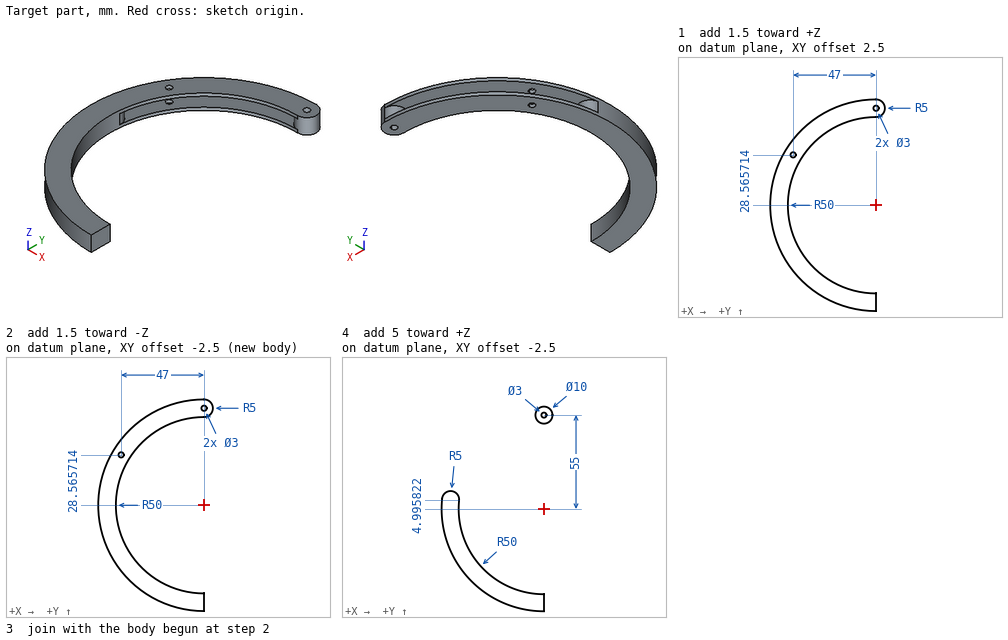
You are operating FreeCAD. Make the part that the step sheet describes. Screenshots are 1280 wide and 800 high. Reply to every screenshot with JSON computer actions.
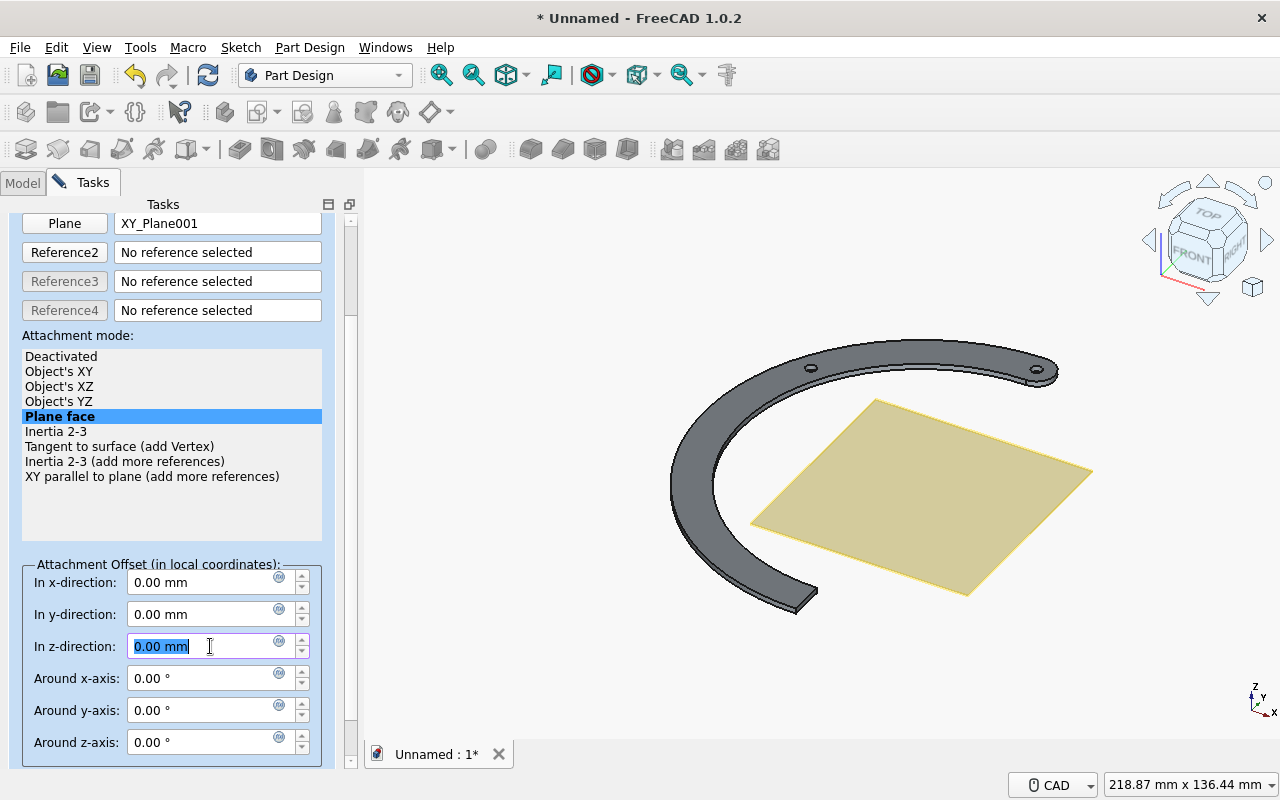
{"action": "type", "text": "-2.5"}
{"action": "key", "text": "Tab"}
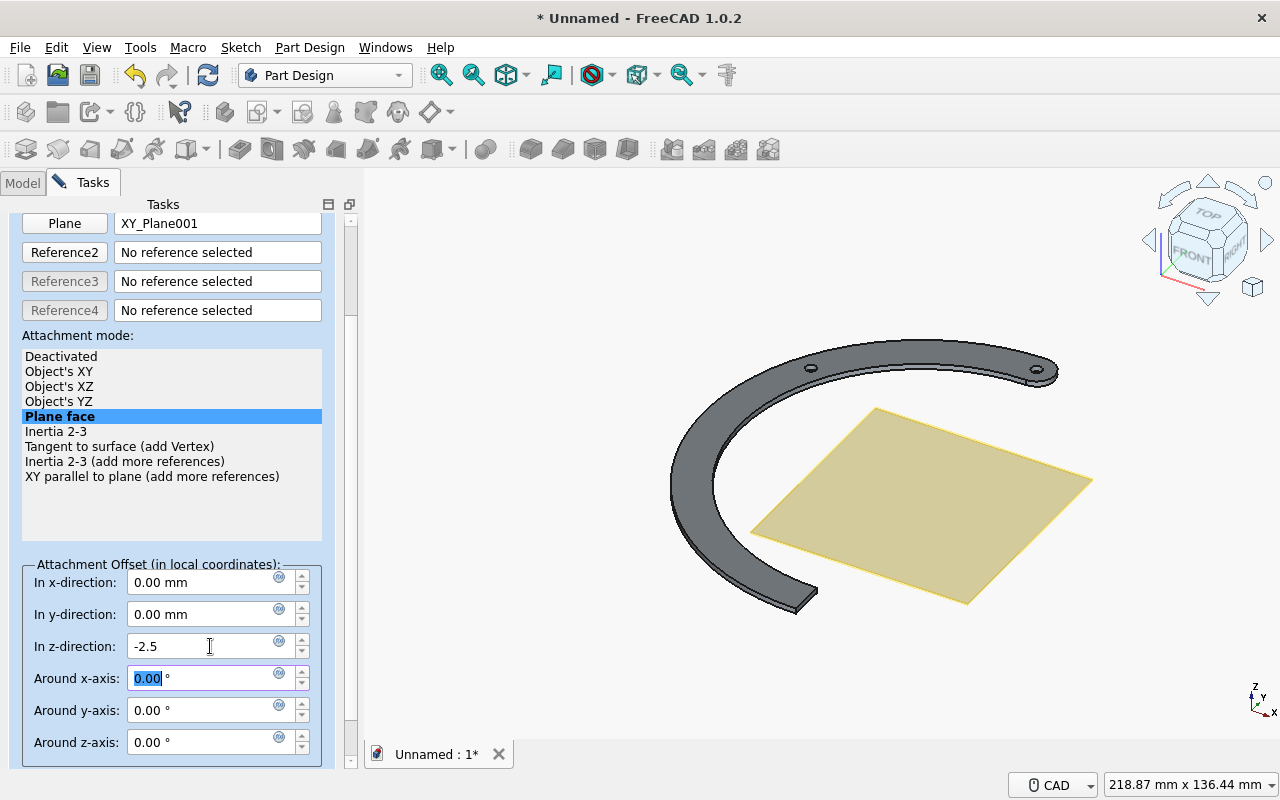
{"action": "scroll", "coordinate": [351, 491], "scroll_direction": "up", "scroll_amount": 3}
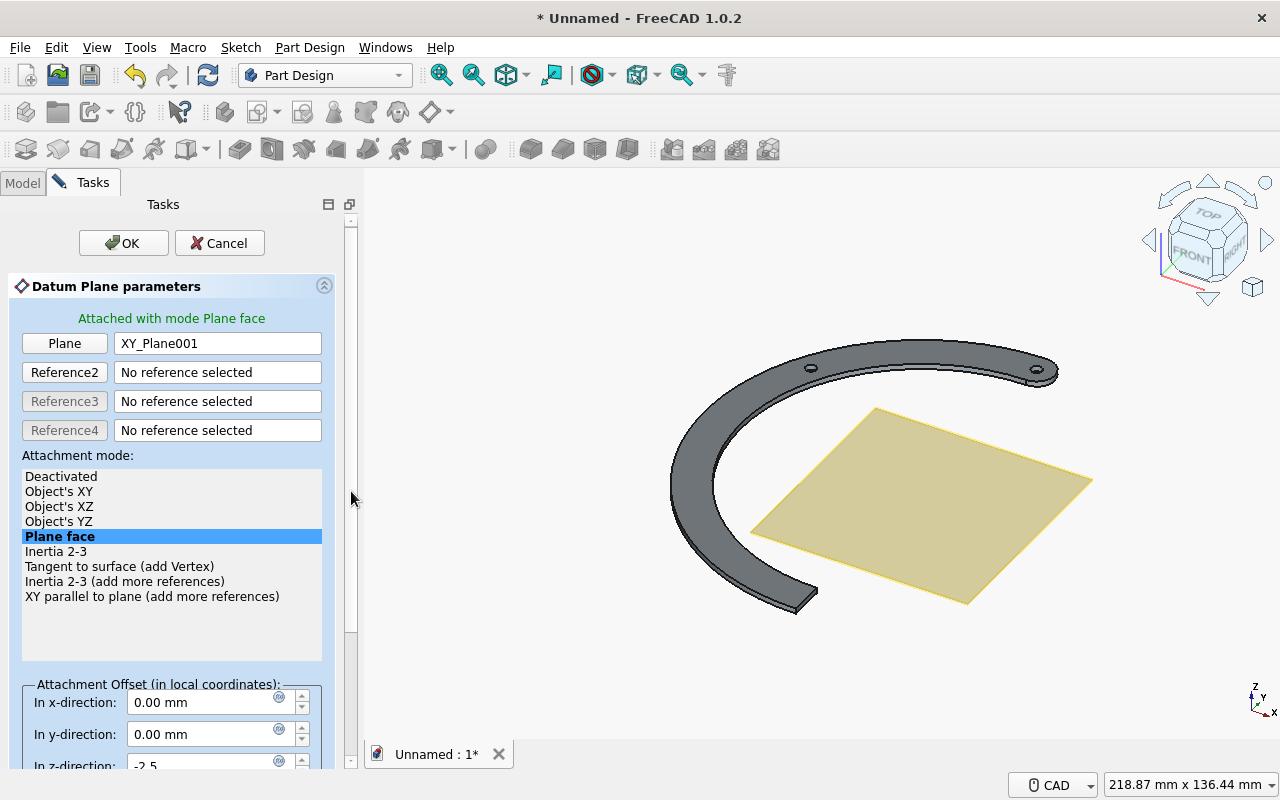
{"action": "left_click", "coordinate": [124, 243]}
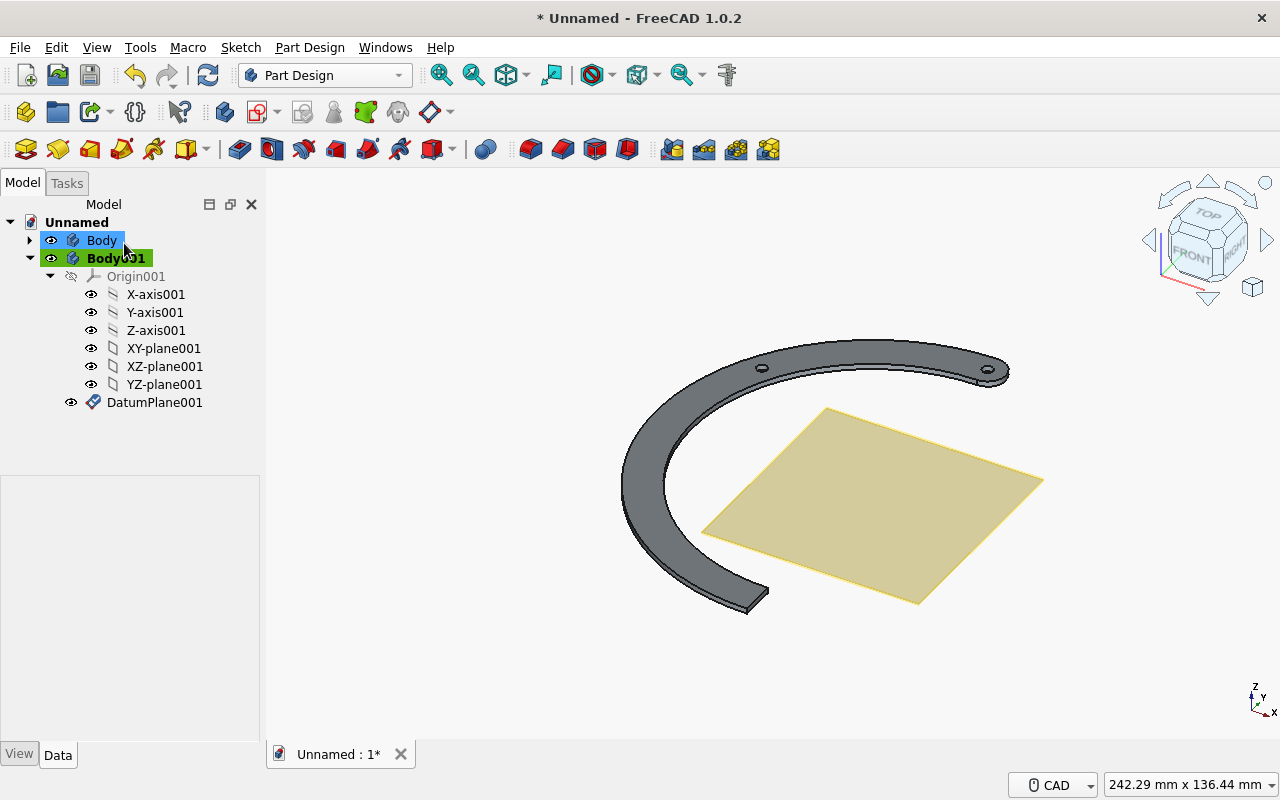
{"action": "left_click", "coordinate": [116, 402]}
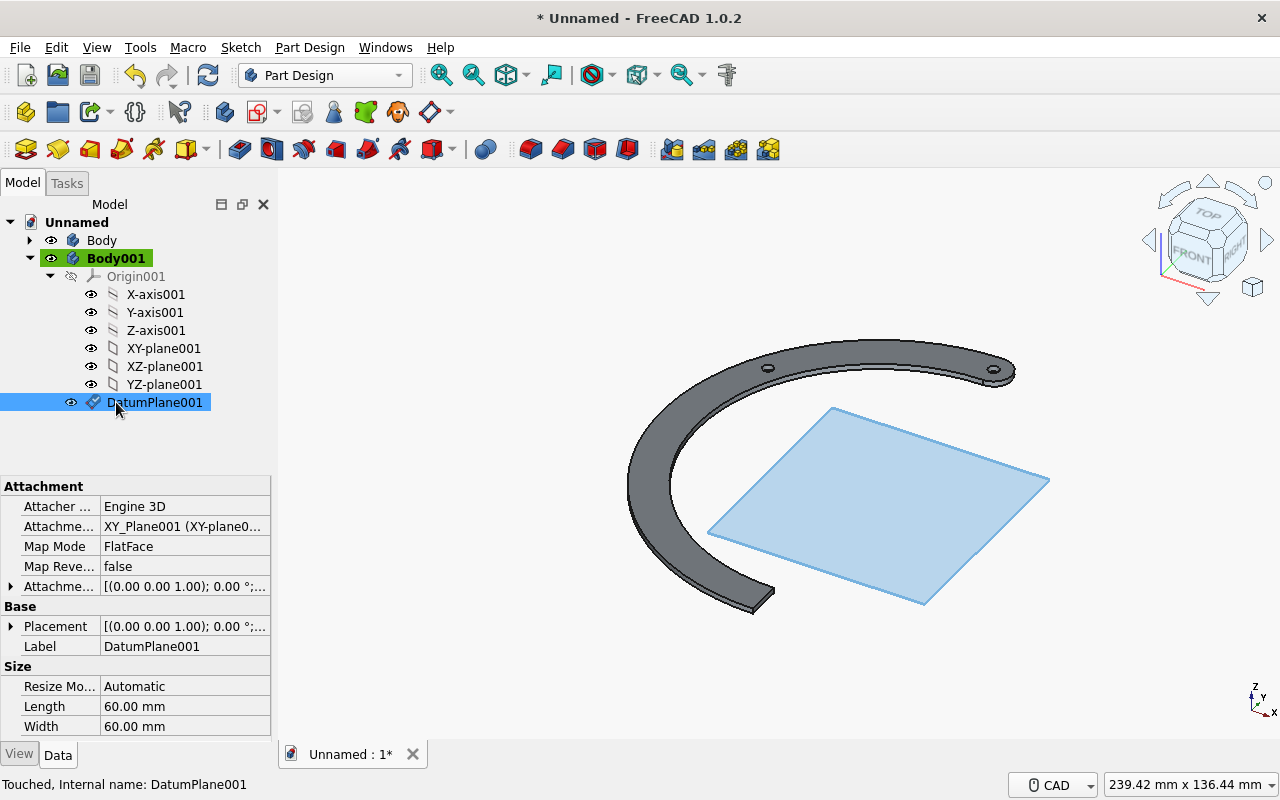
{"action": "left_click", "coordinate": [258, 112]}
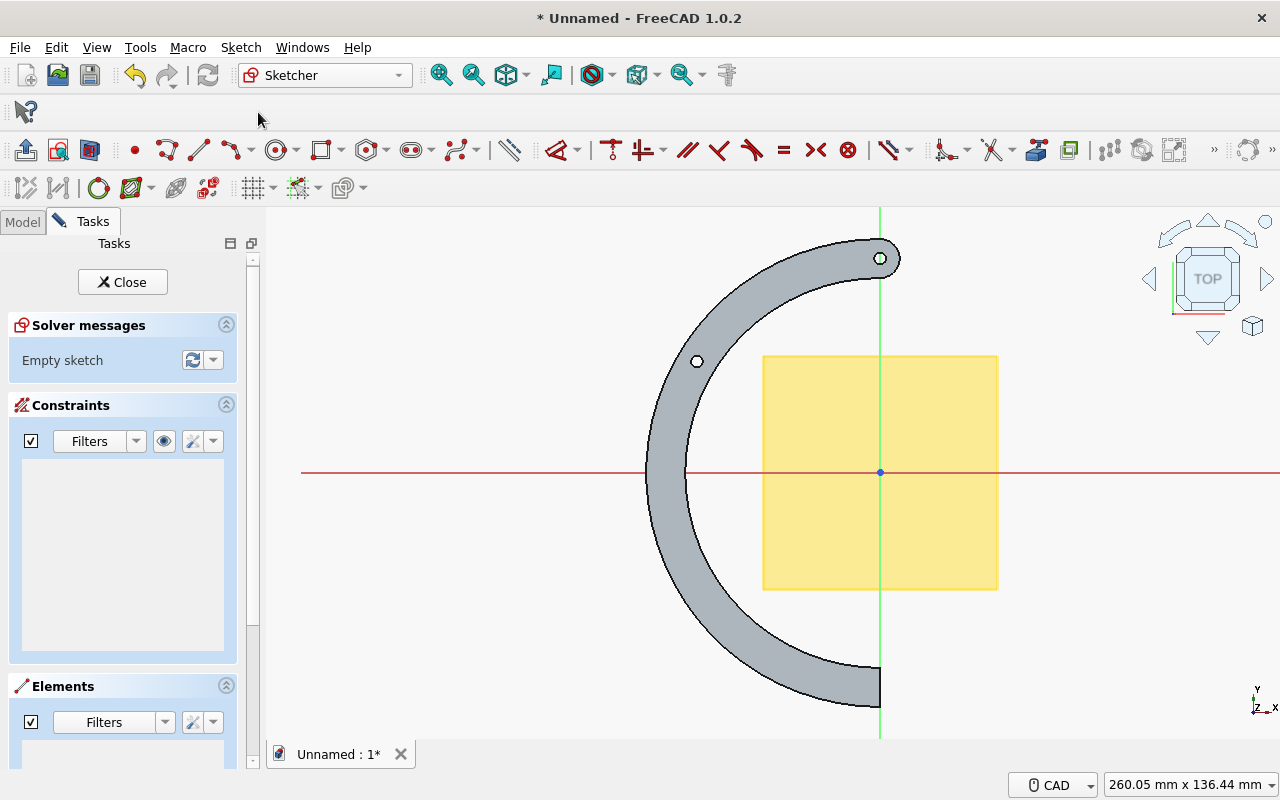
{"action": "scroll", "coordinate": [565, 473], "scroll_direction": "down", "scroll_amount": 2}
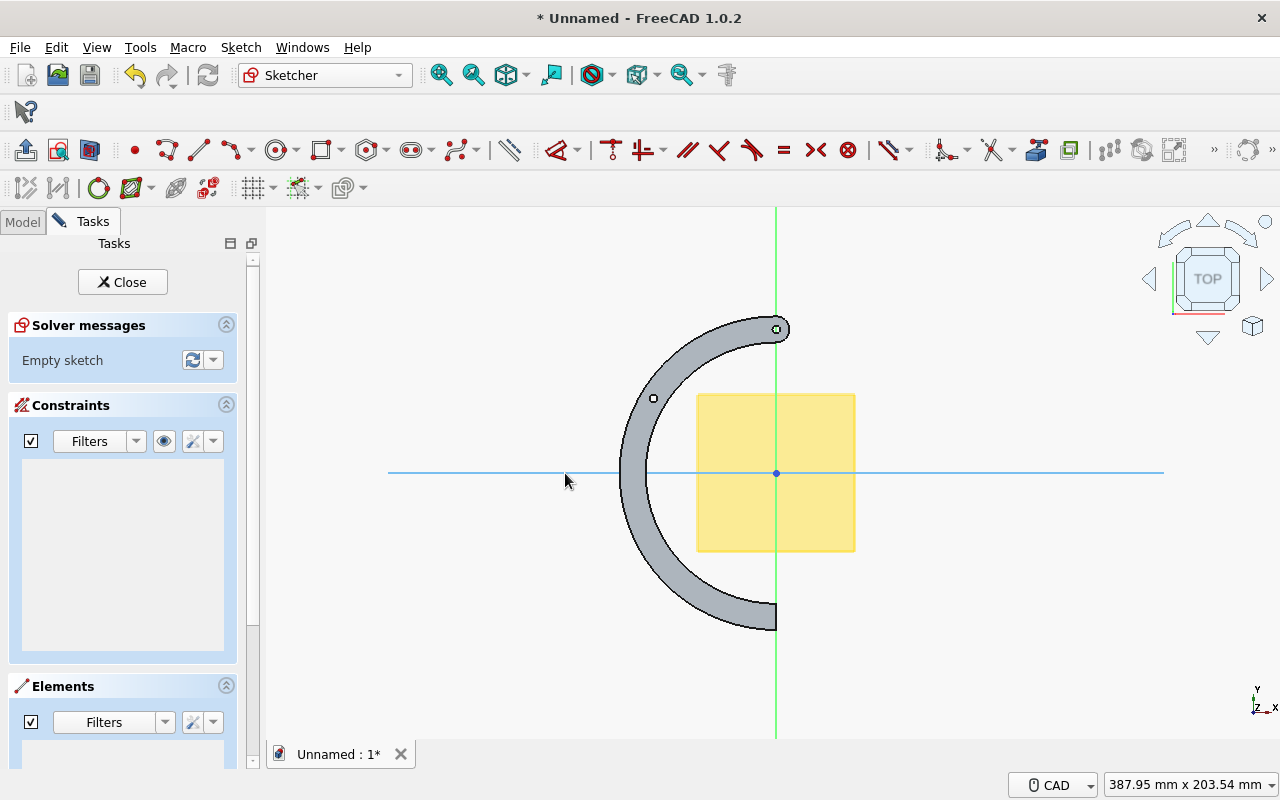
{"action": "left_click", "coordinate": [200, 150]}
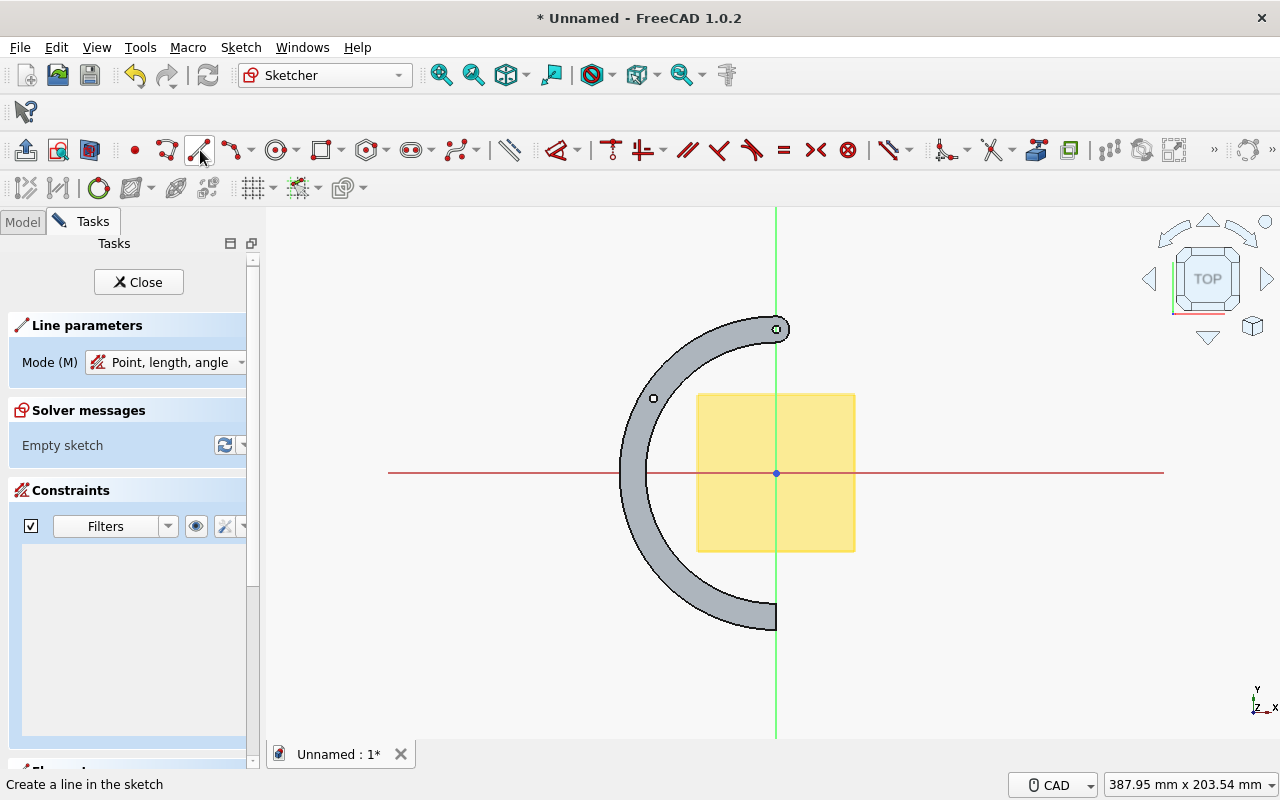
{"action": "left_click", "coordinate": [776, 630]}
{"action": "left_click", "coordinate": [767, 604]}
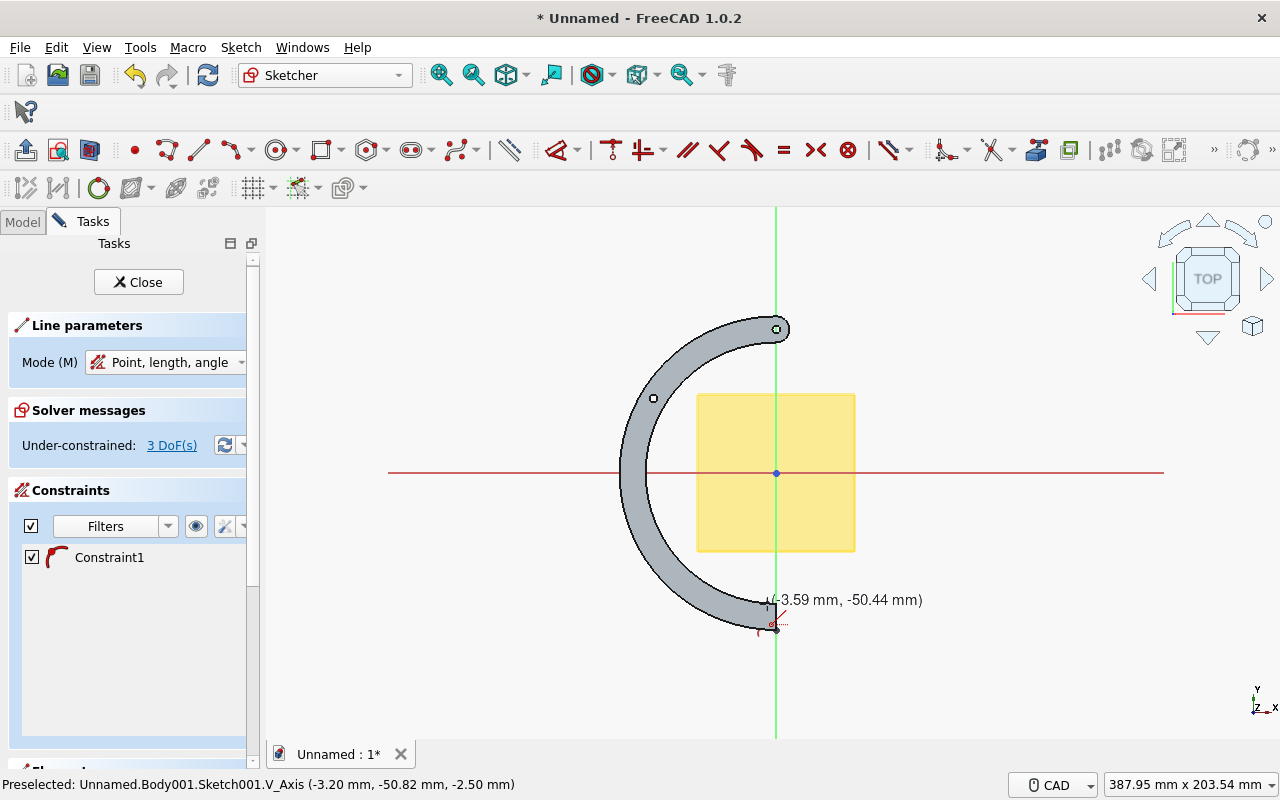
{"action": "left_click", "coordinate": [232, 150]}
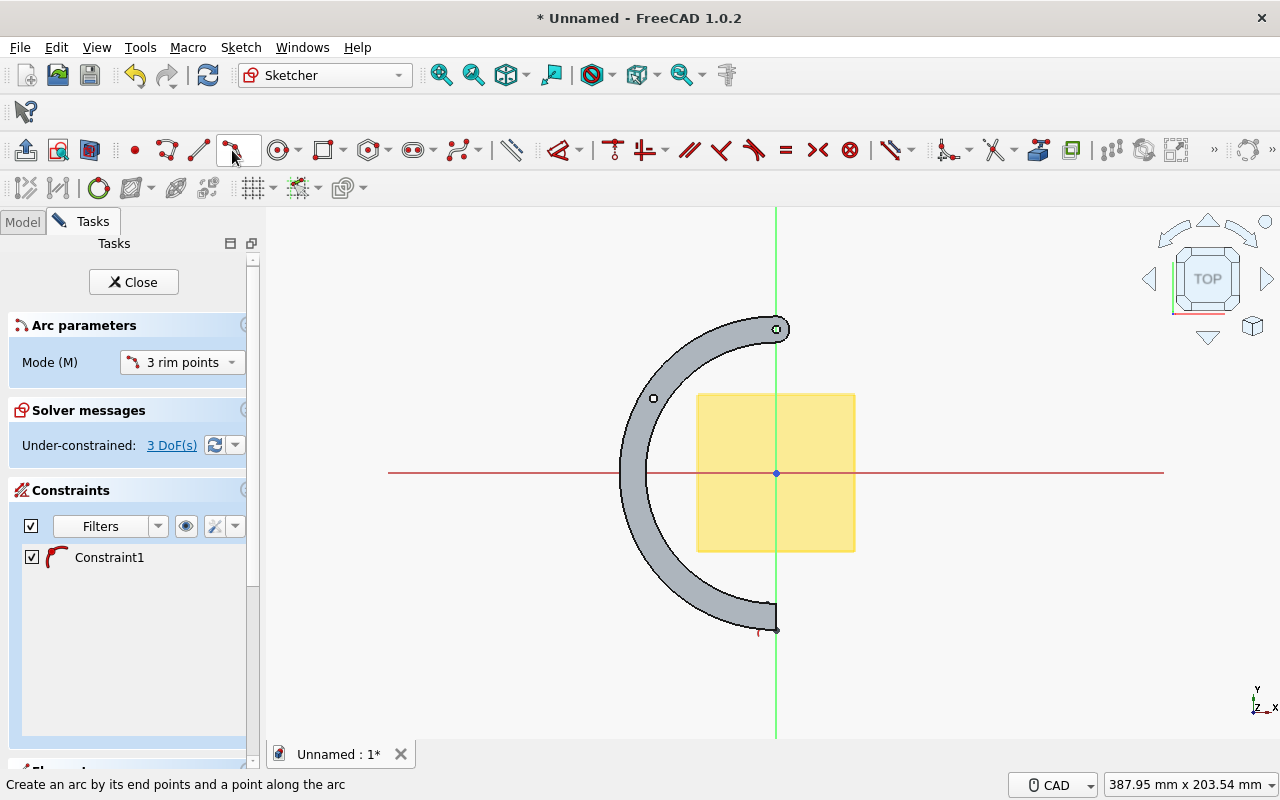
{"action": "left_click", "coordinate": [767, 605]}
{"action": "left_click", "coordinate": [776, 342]}
{"action": "left_click", "coordinate": [652, 433]}